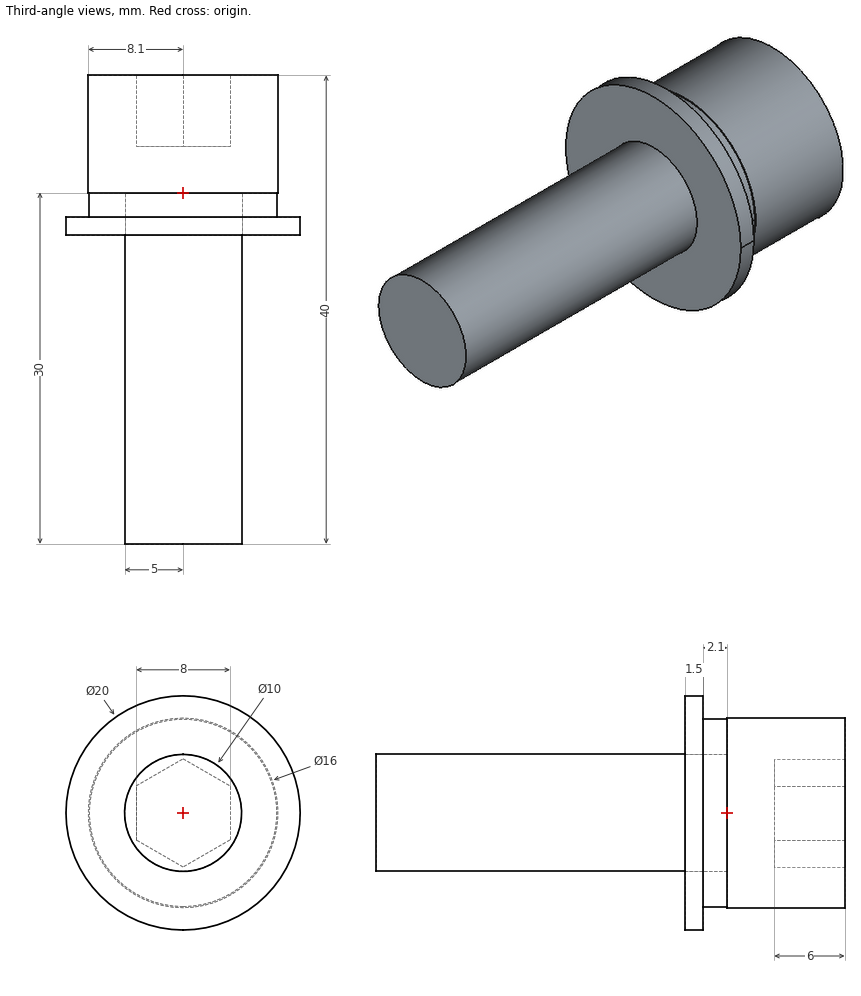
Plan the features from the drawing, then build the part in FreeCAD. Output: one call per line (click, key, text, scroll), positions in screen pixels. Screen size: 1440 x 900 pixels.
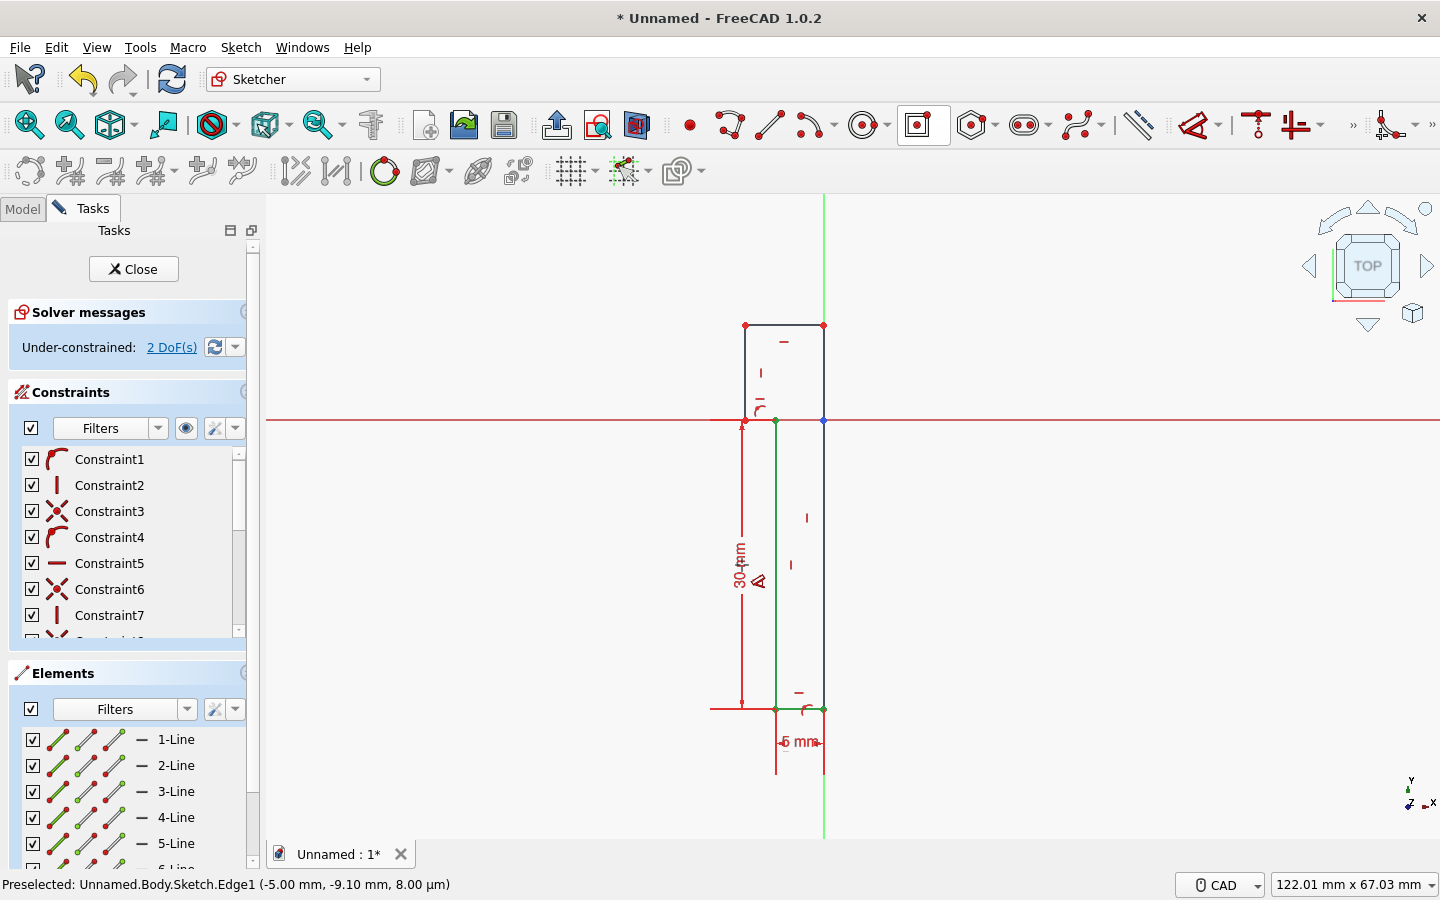
click(824, 594)
click(858, 517)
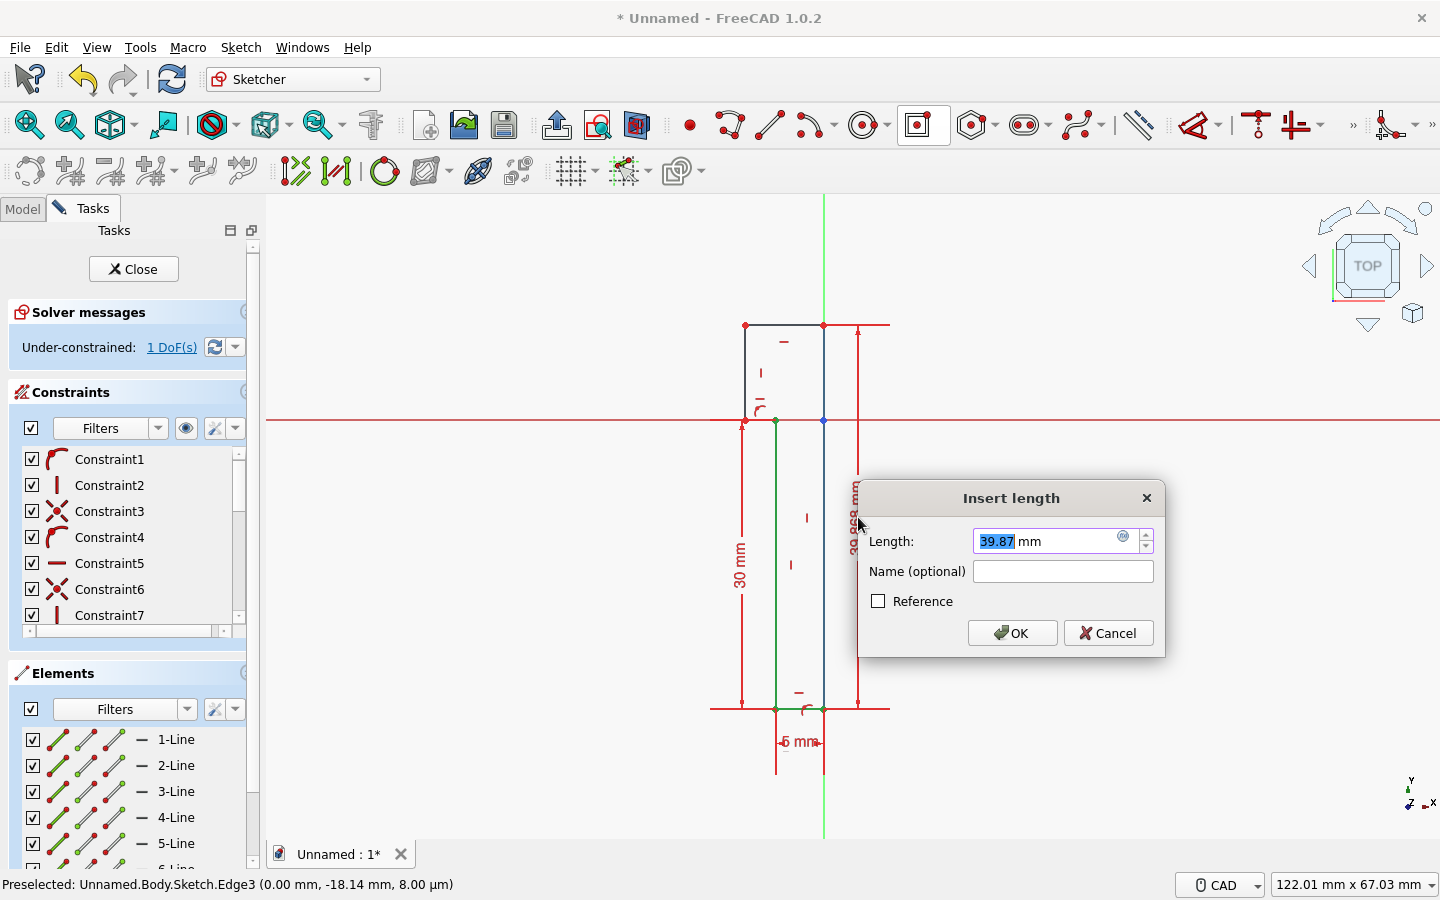
text(40)
key(Return)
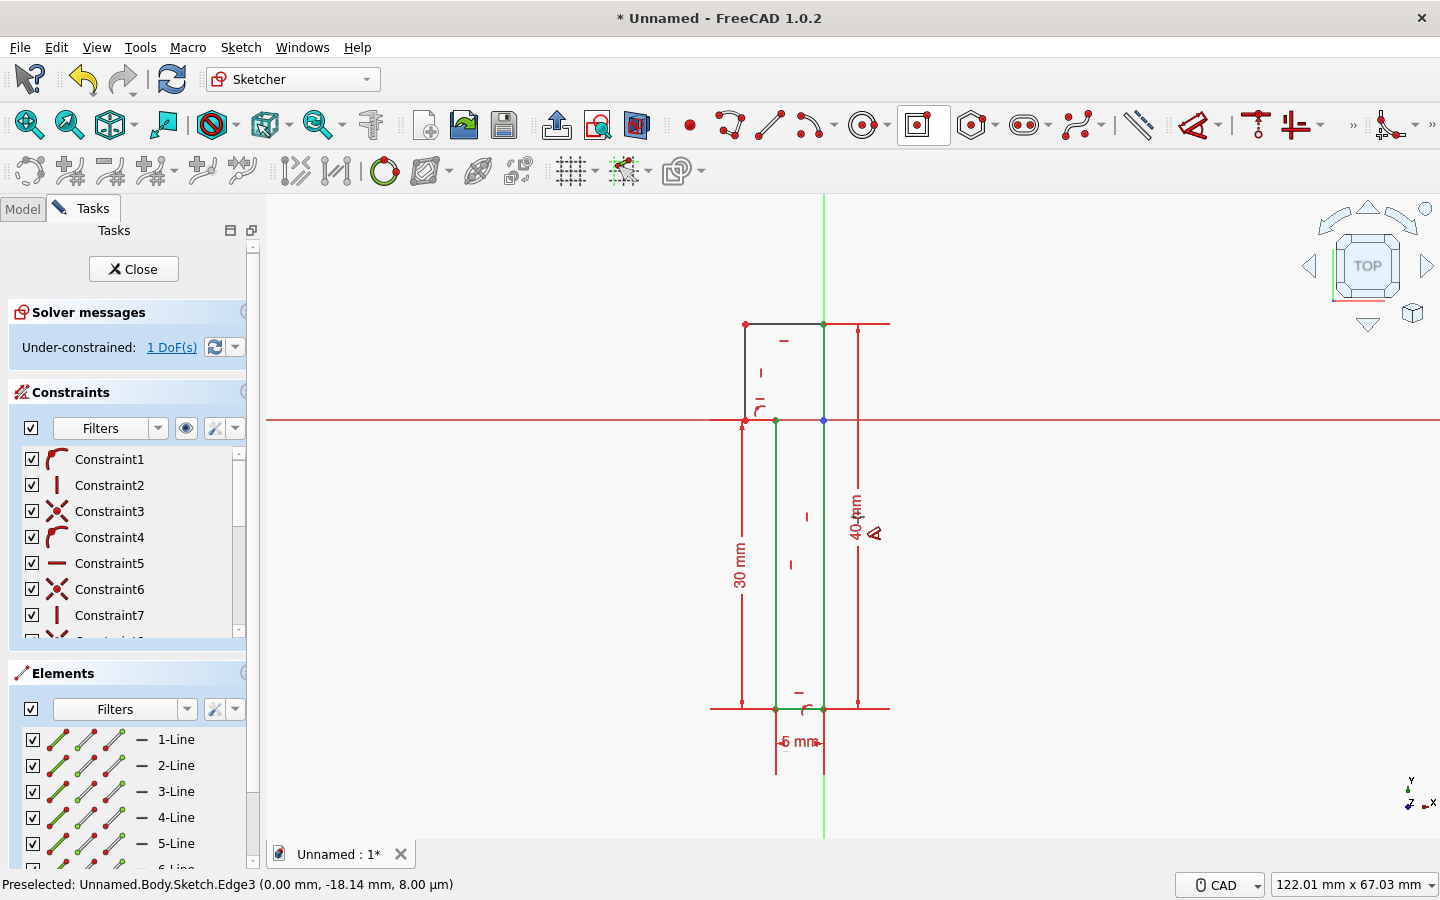
click(800, 324)
click(785, 290)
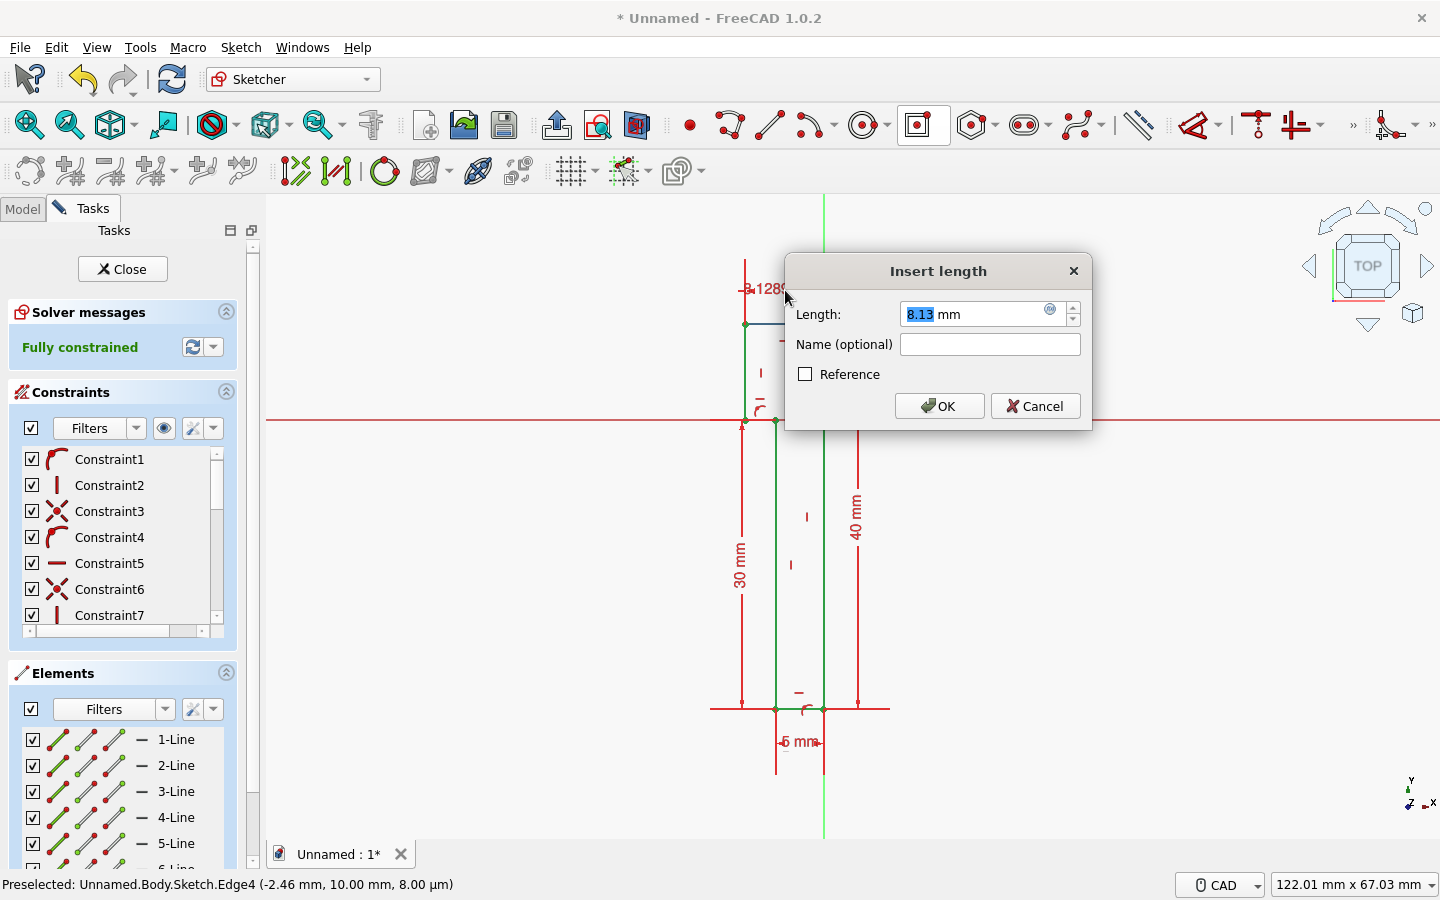
text(8.1)
key(Return)
key(Escape)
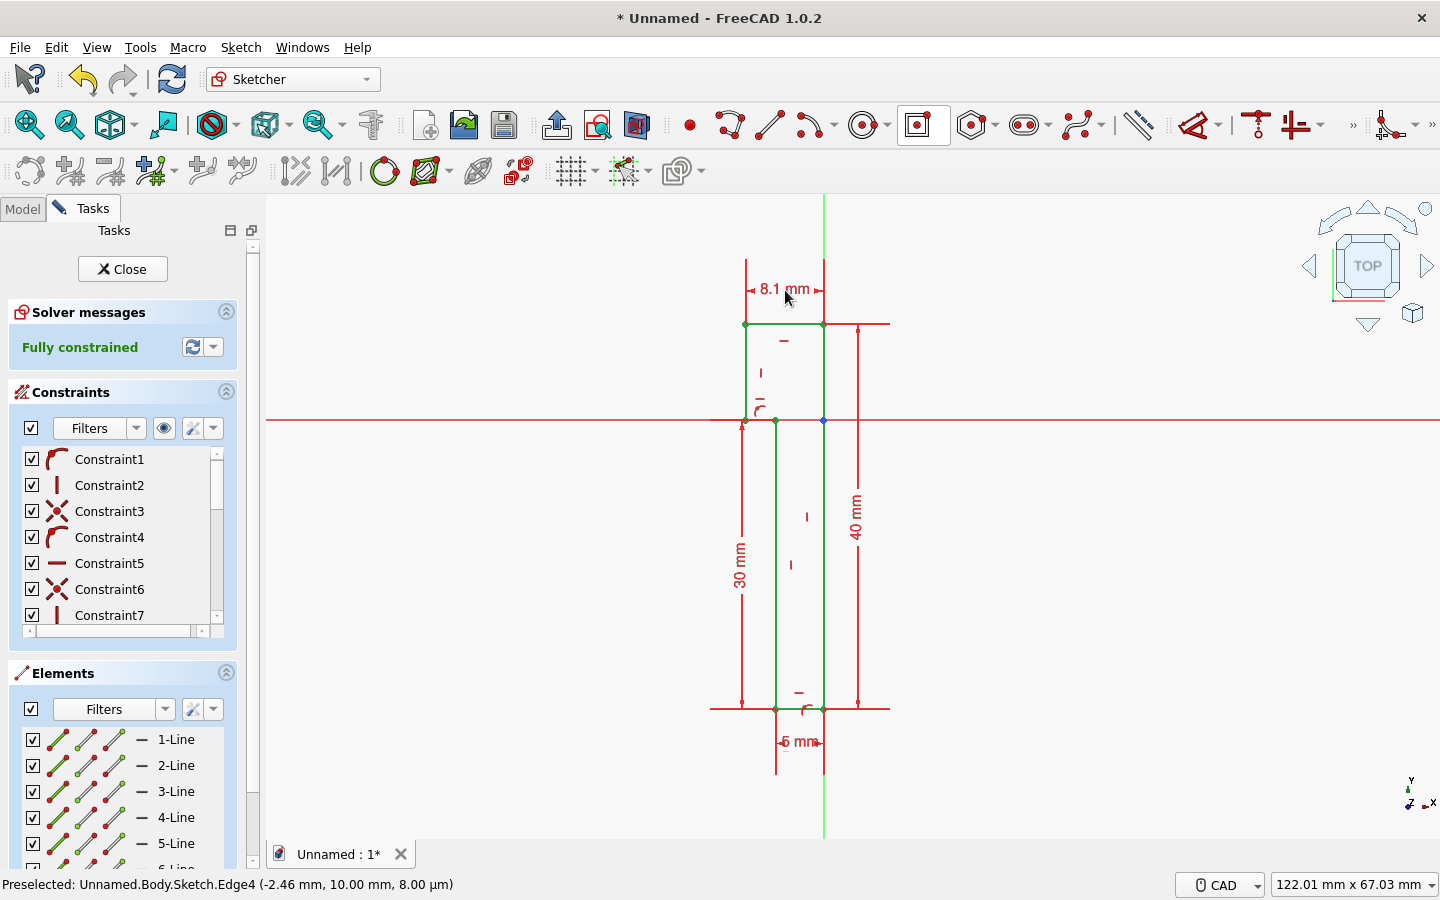
click(123, 269)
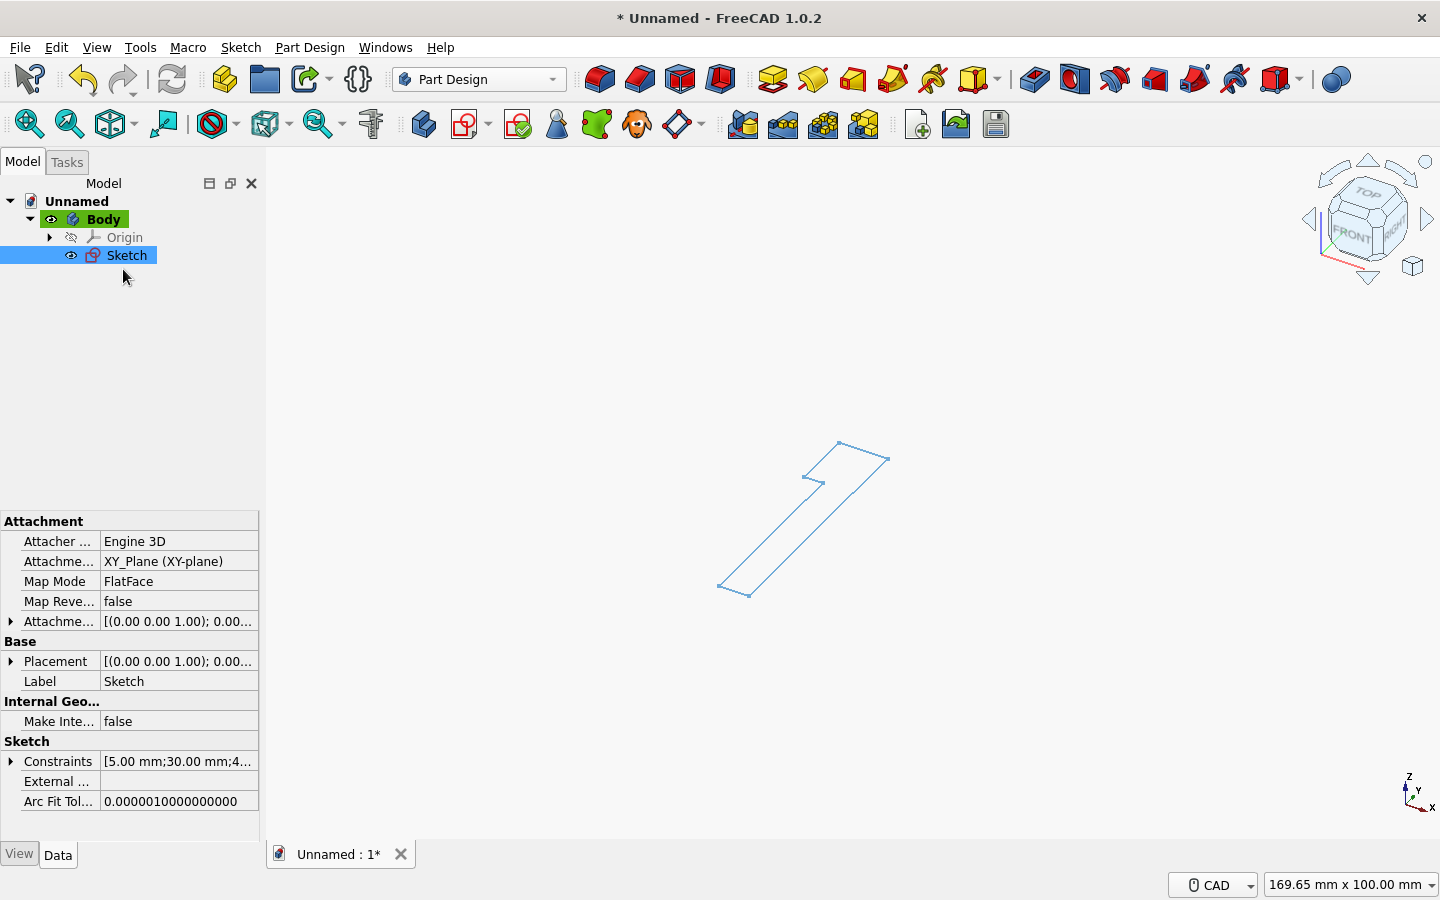
click(814, 80)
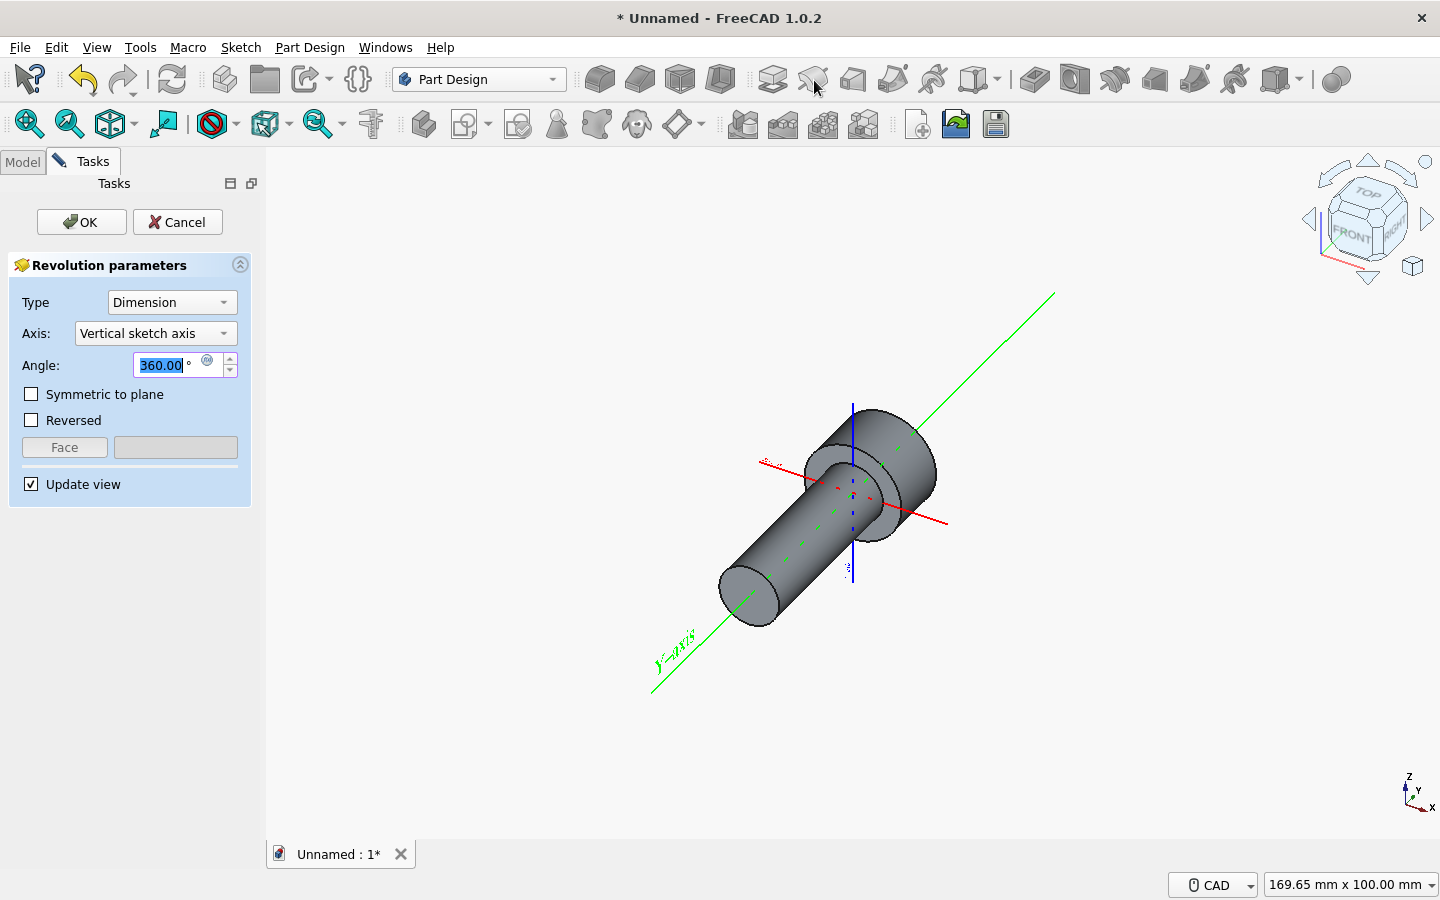
click(82, 222)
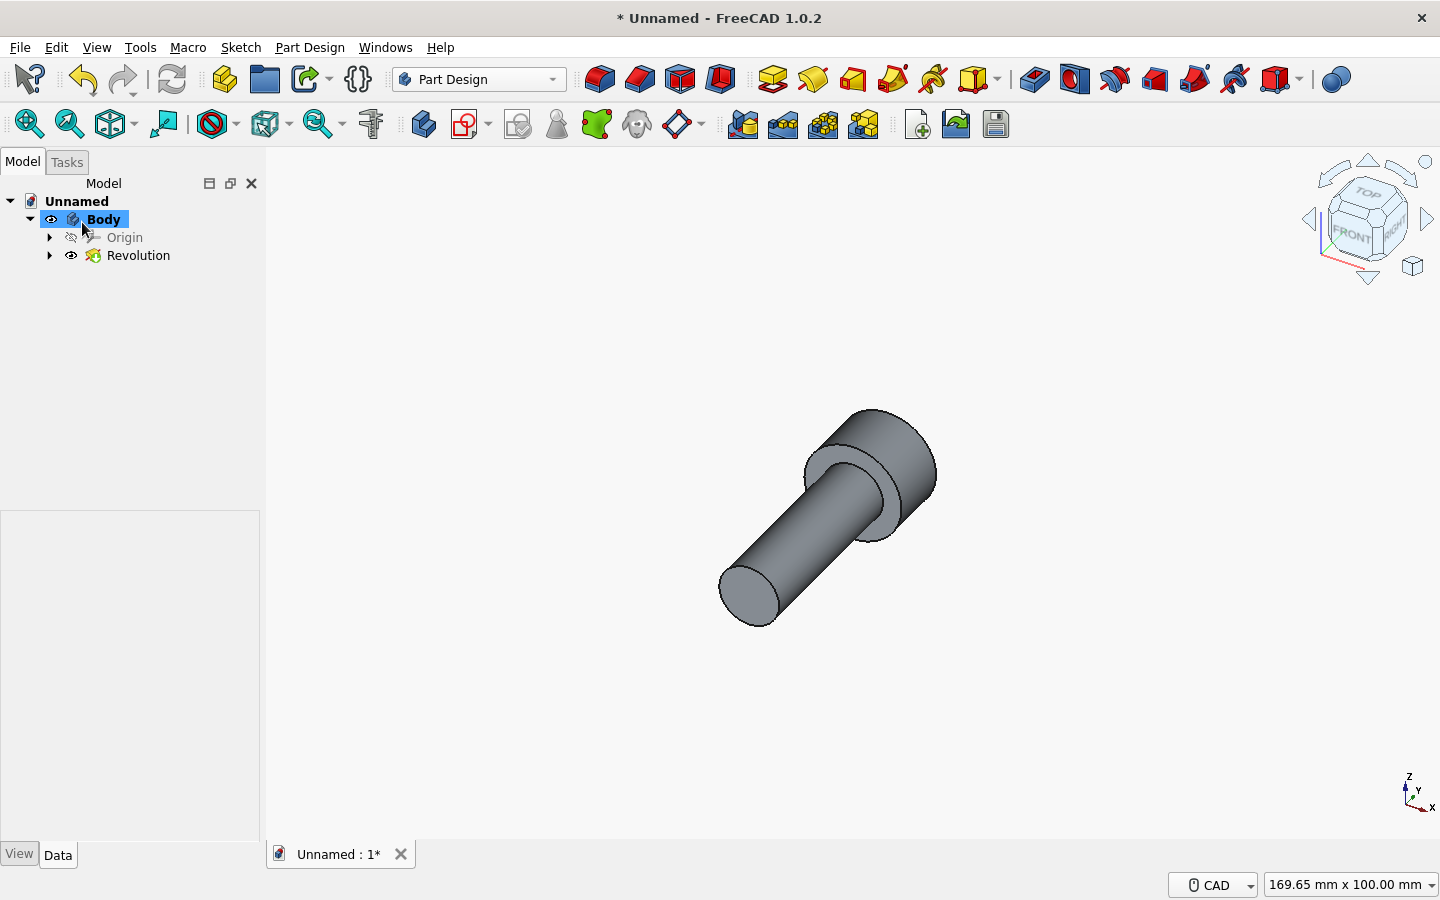
key(v)
key(f)